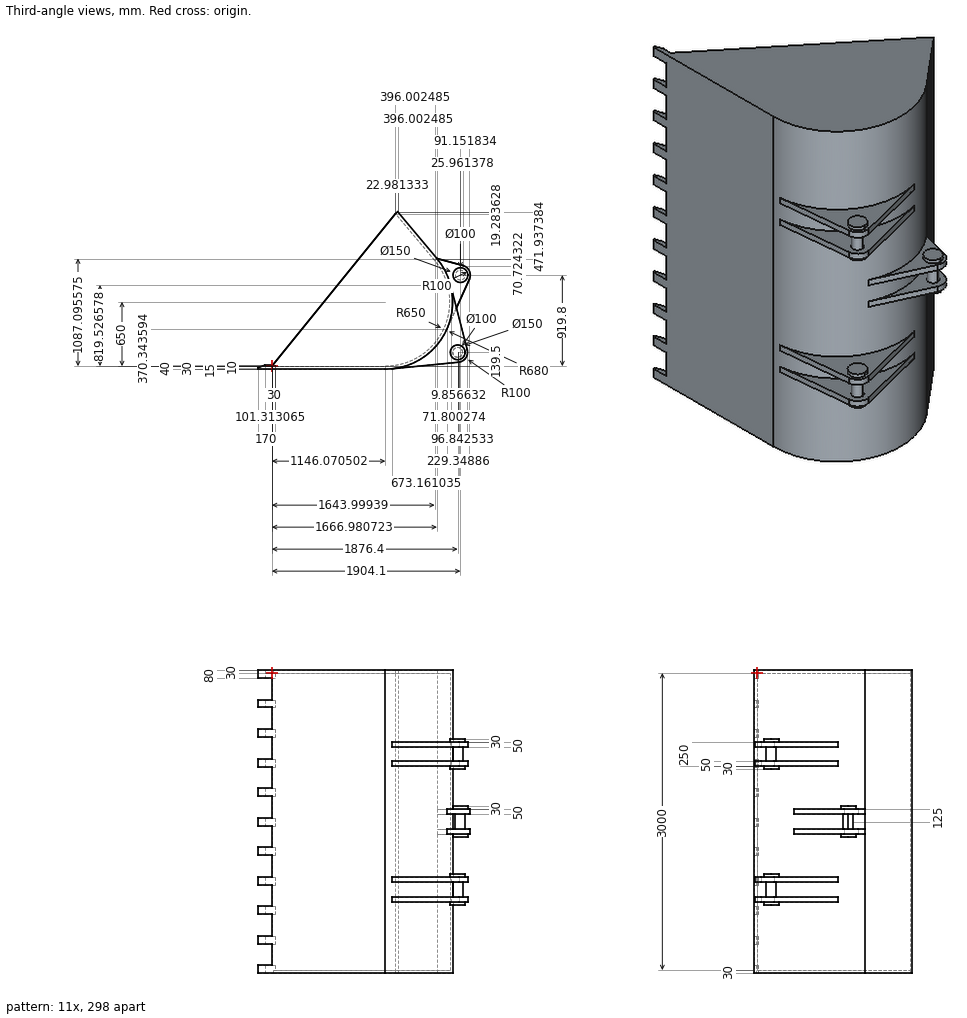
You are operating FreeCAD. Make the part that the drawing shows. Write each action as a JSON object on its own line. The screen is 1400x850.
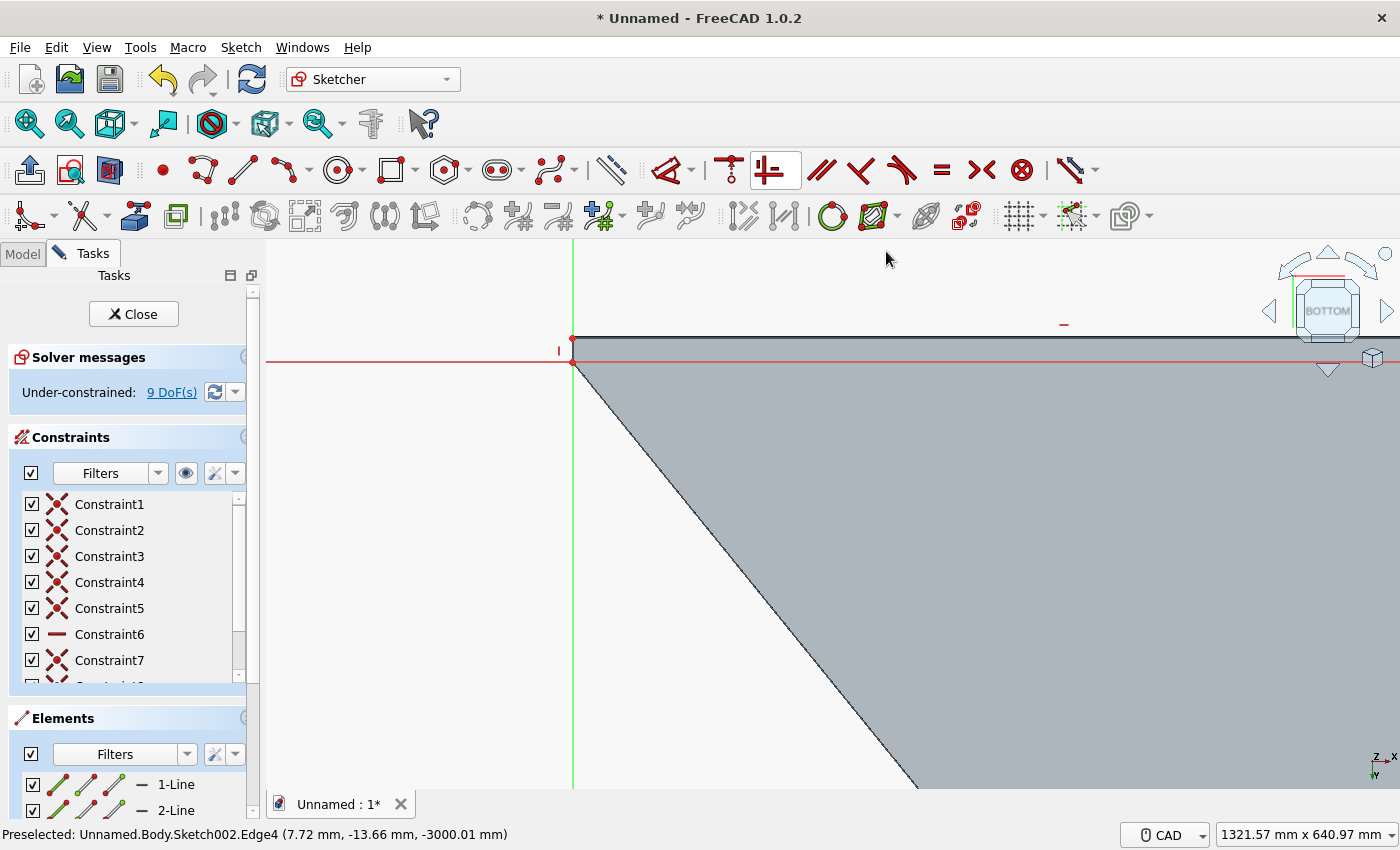
{"action": "left_click", "coordinate": [666, 170]}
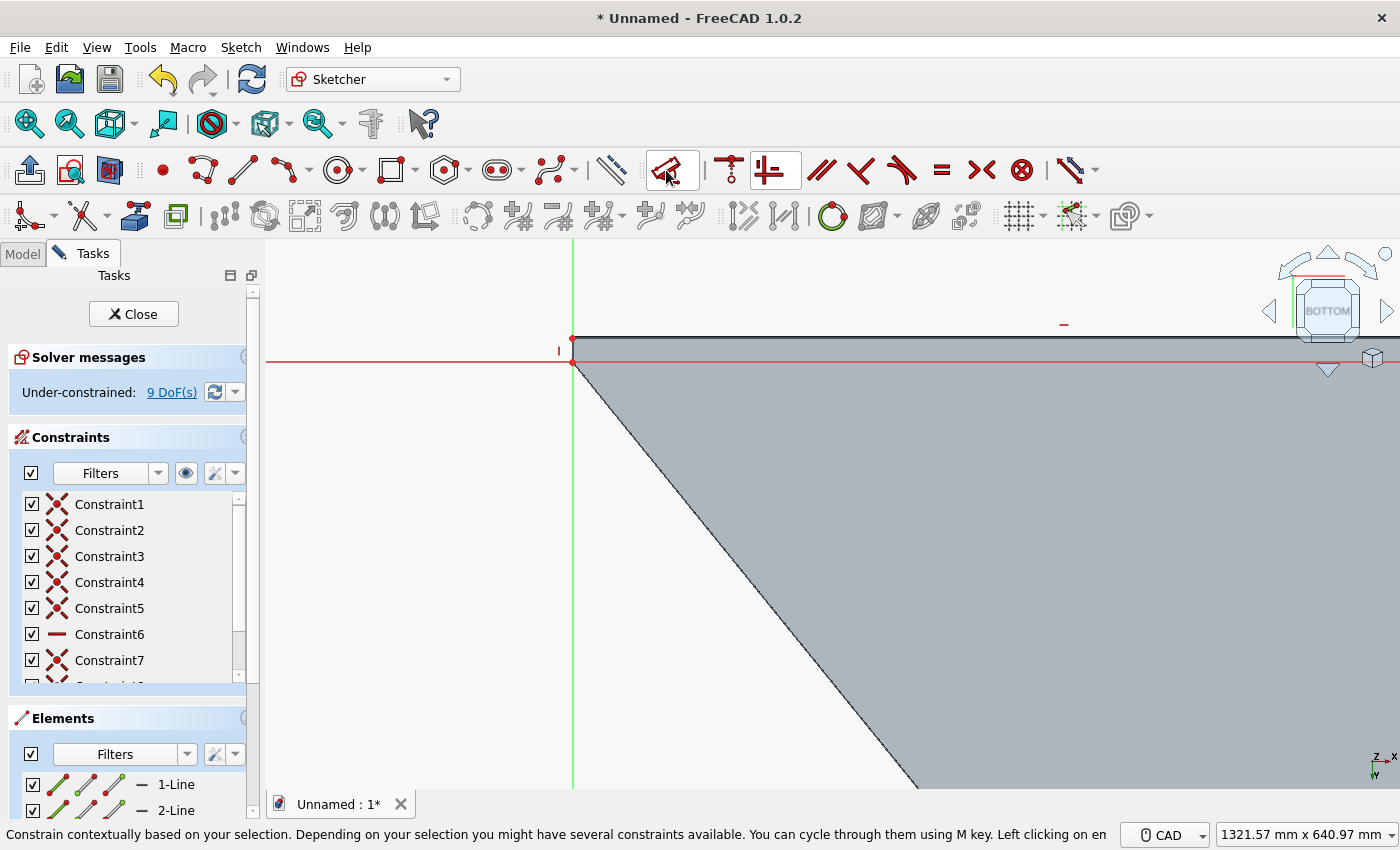
{"action": "scroll", "coordinate": [580, 349], "scroll_direction": "down", "scroll_amount": 7}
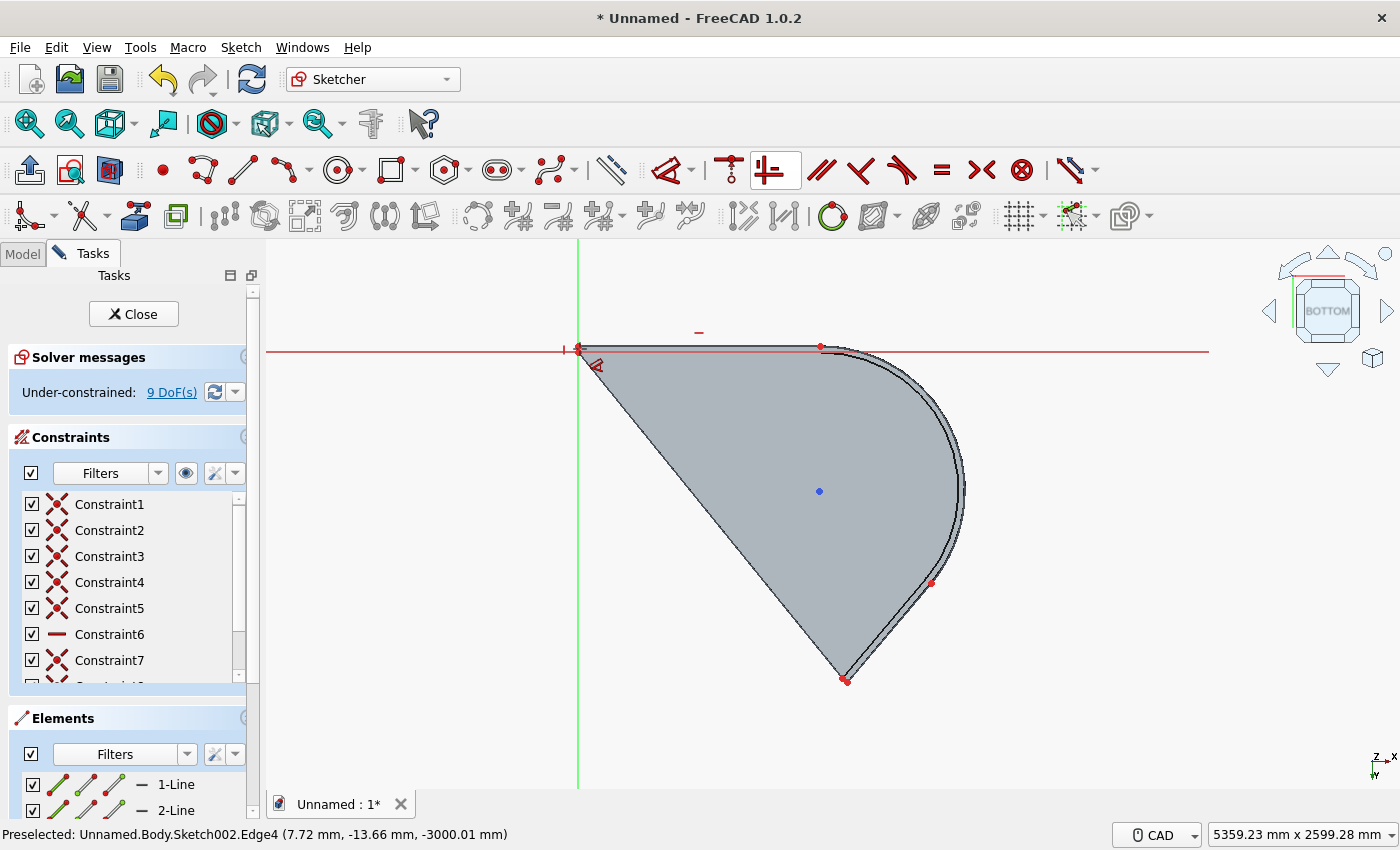
{"action": "left_click", "coordinate": [965, 494]}
{"action": "left_click", "coordinate": [997, 495]}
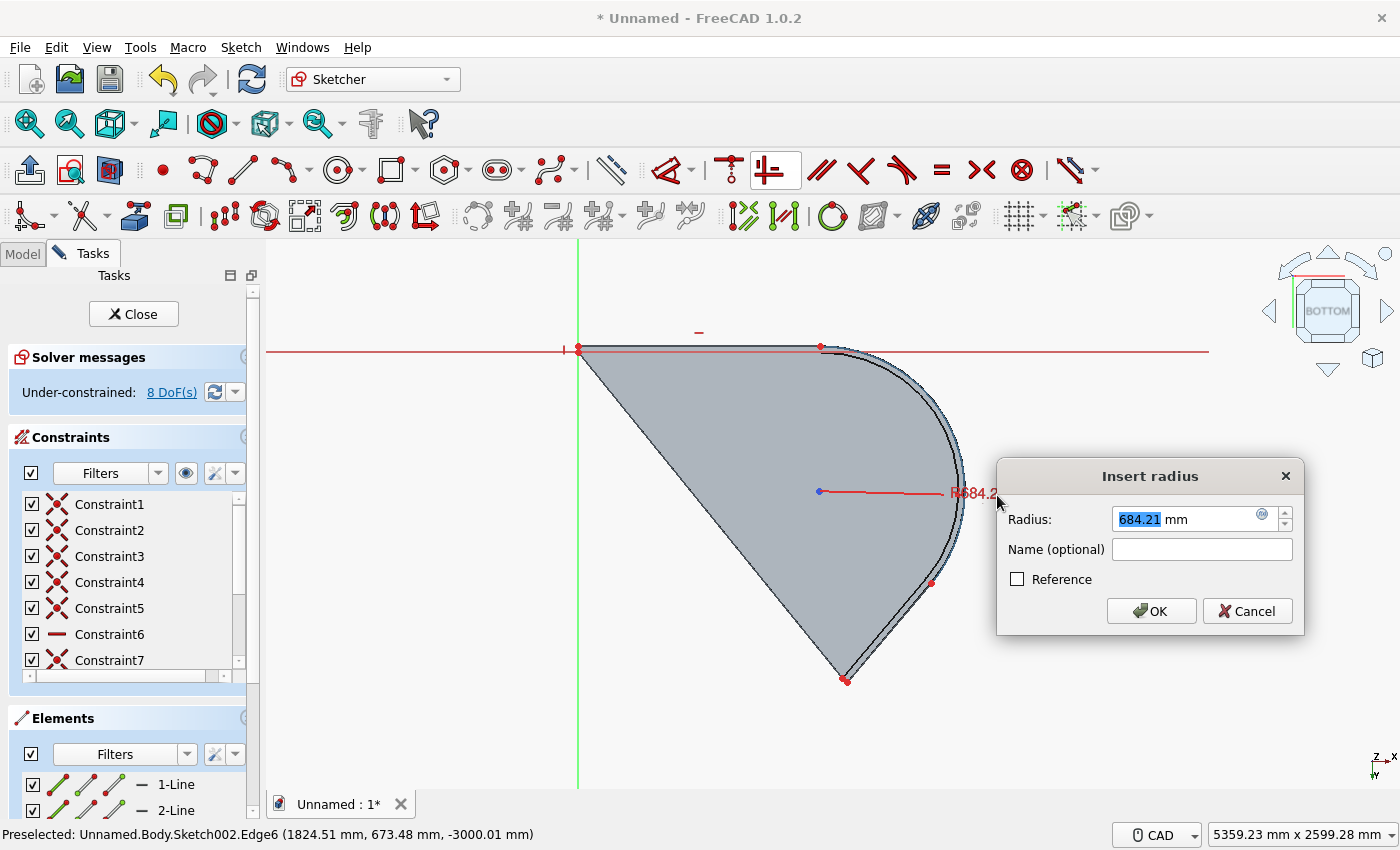
{"action": "type", "text": "680"}
{"action": "key", "text": "Return"}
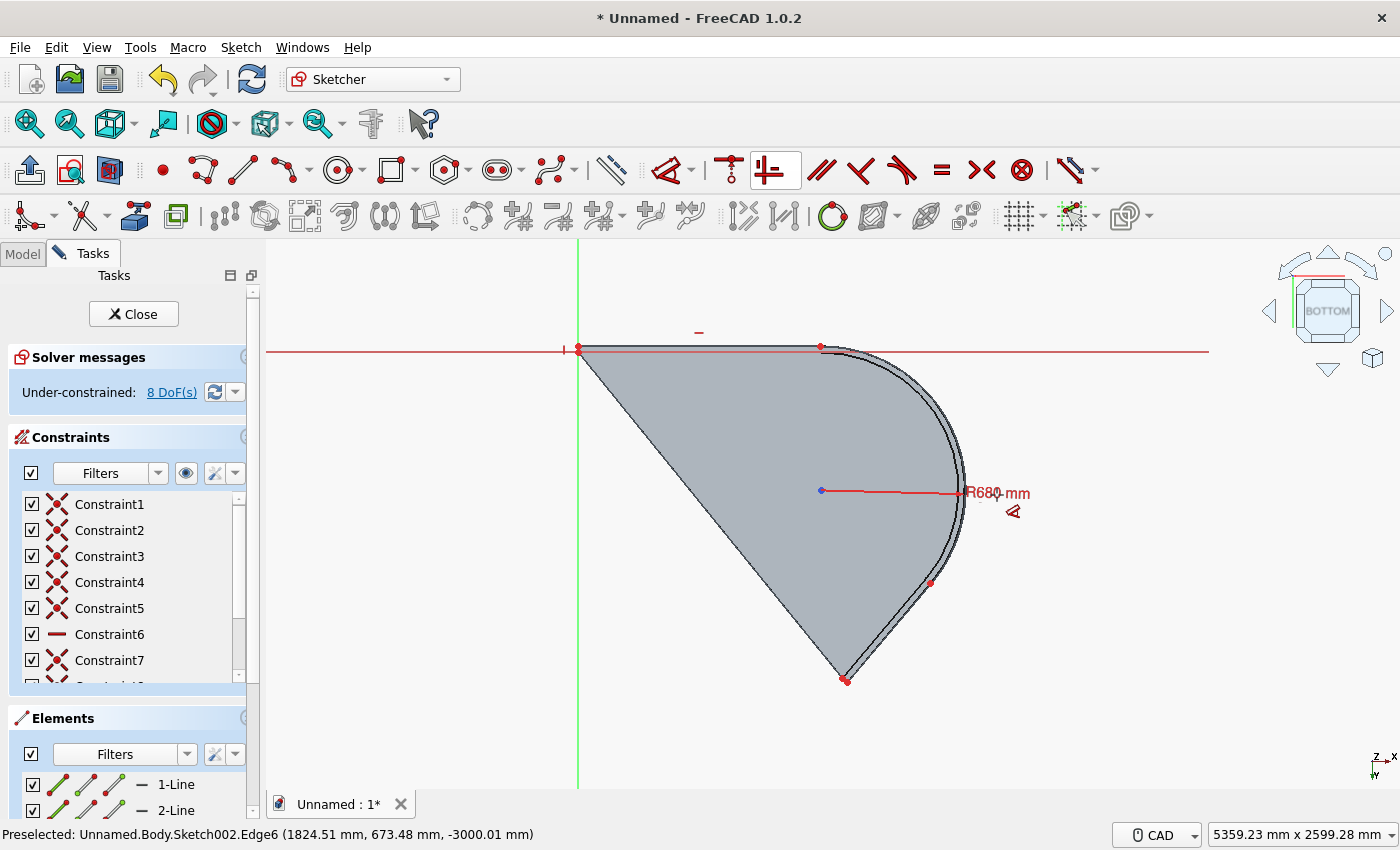
{"action": "scroll", "coordinate": [578, 349], "scroll_direction": "up", "scroll_amount": 10}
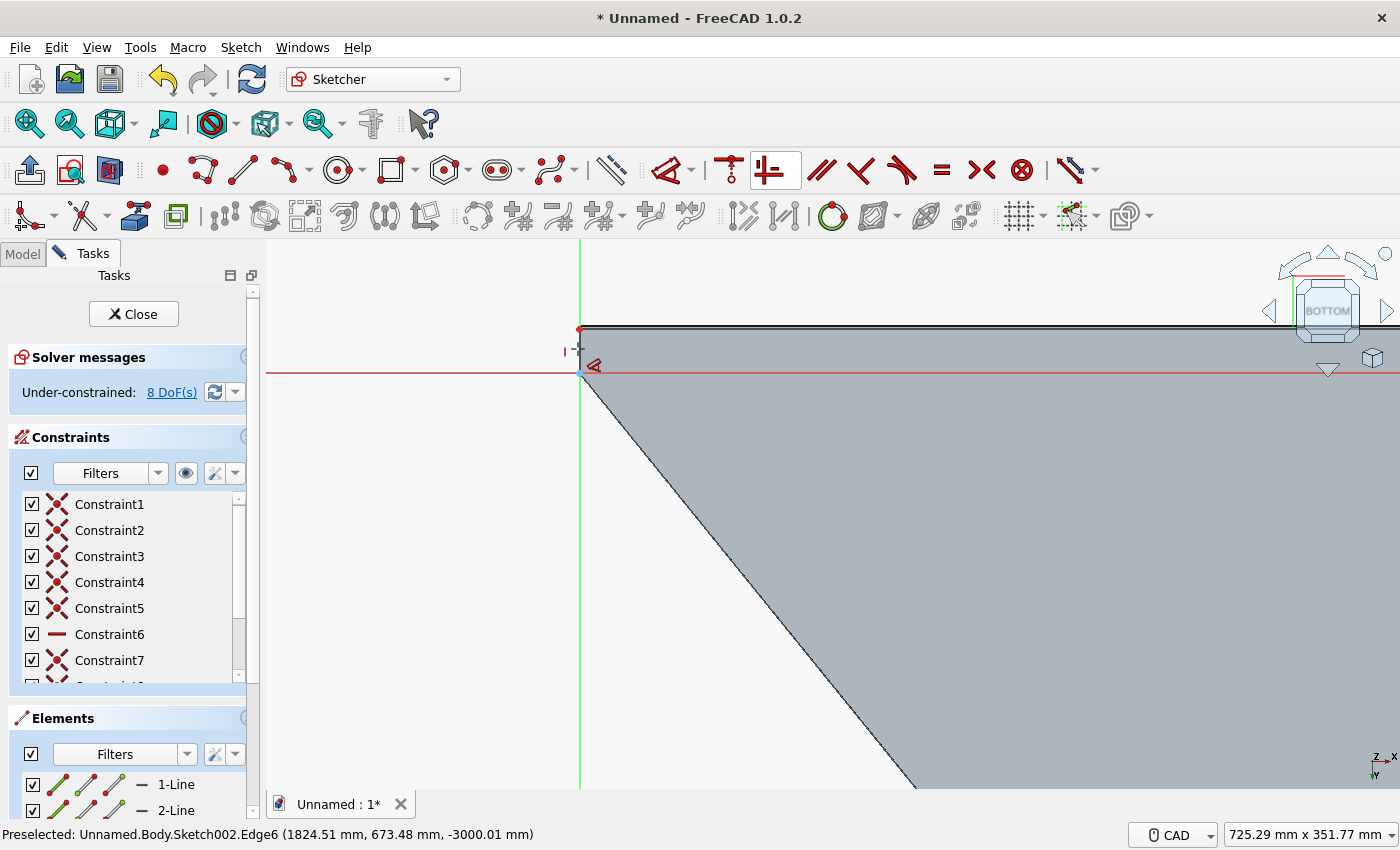
{"action": "left_click", "coordinate": [580, 351]}
{"action": "left_click", "coordinate": [546, 351]}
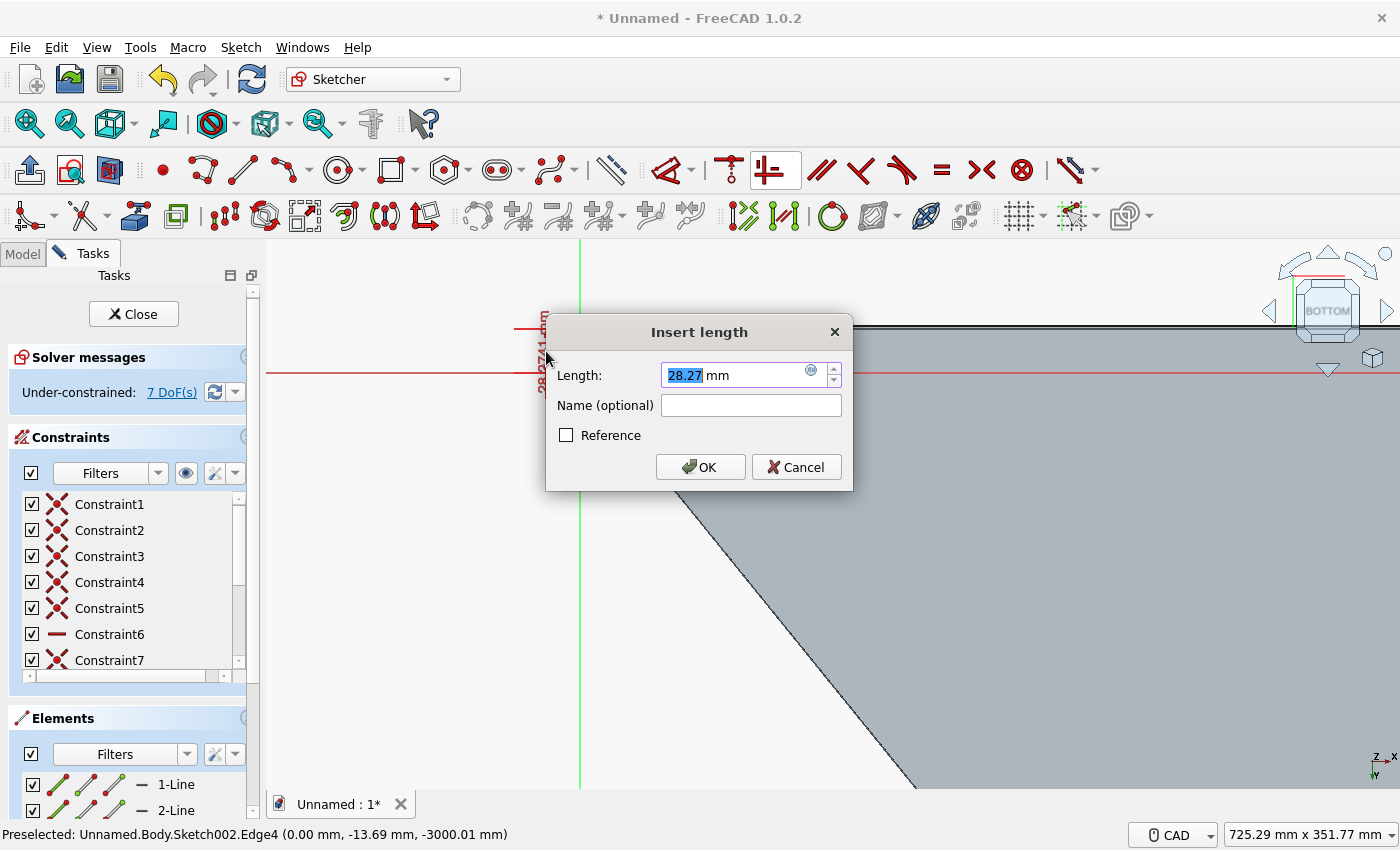
{"action": "type", "text": "30"}
{"action": "key", "text": "Return"}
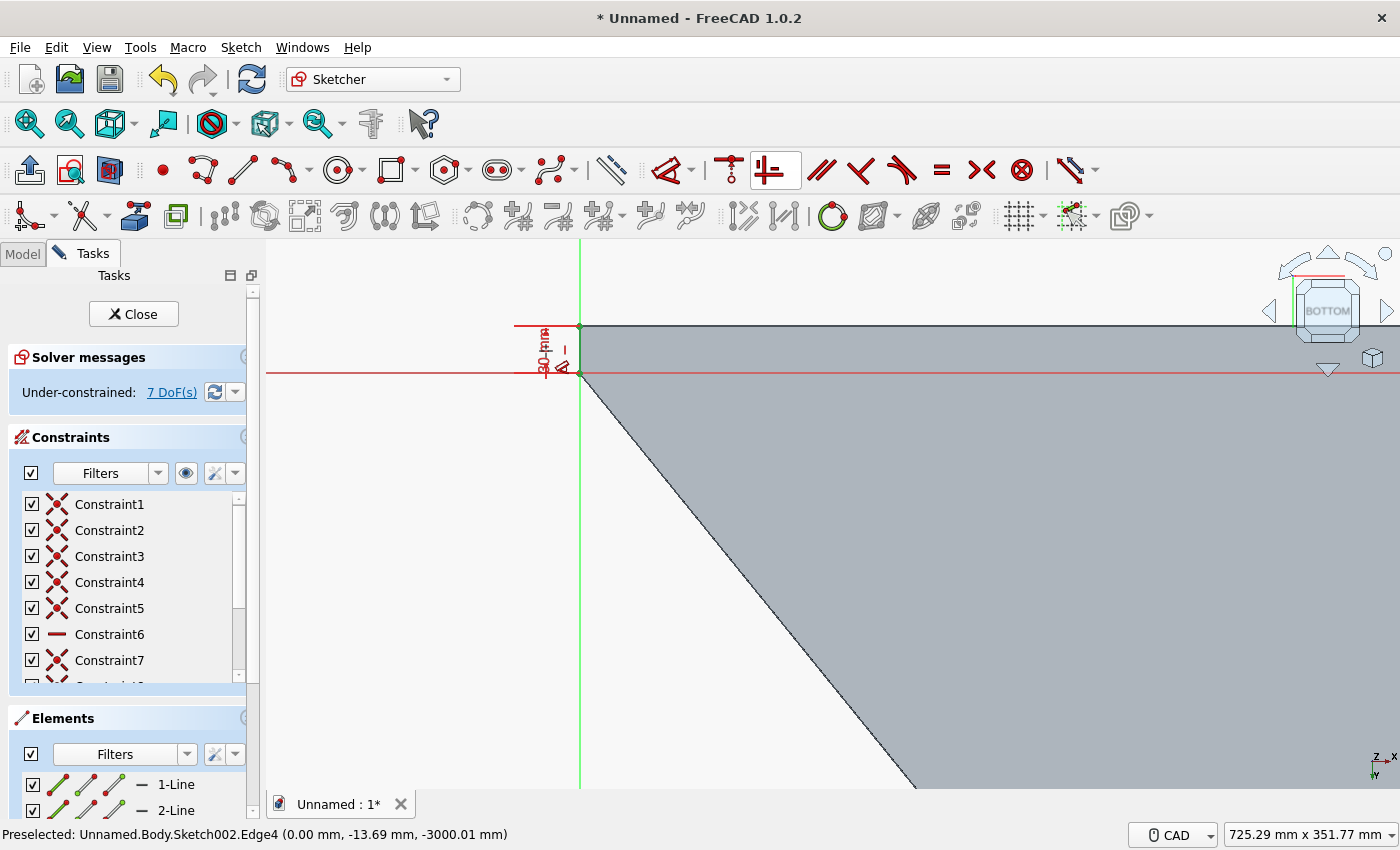
{"action": "scroll", "coordinate": [578, 349], "scroll_direction": "down", "scroll_amount": 10}